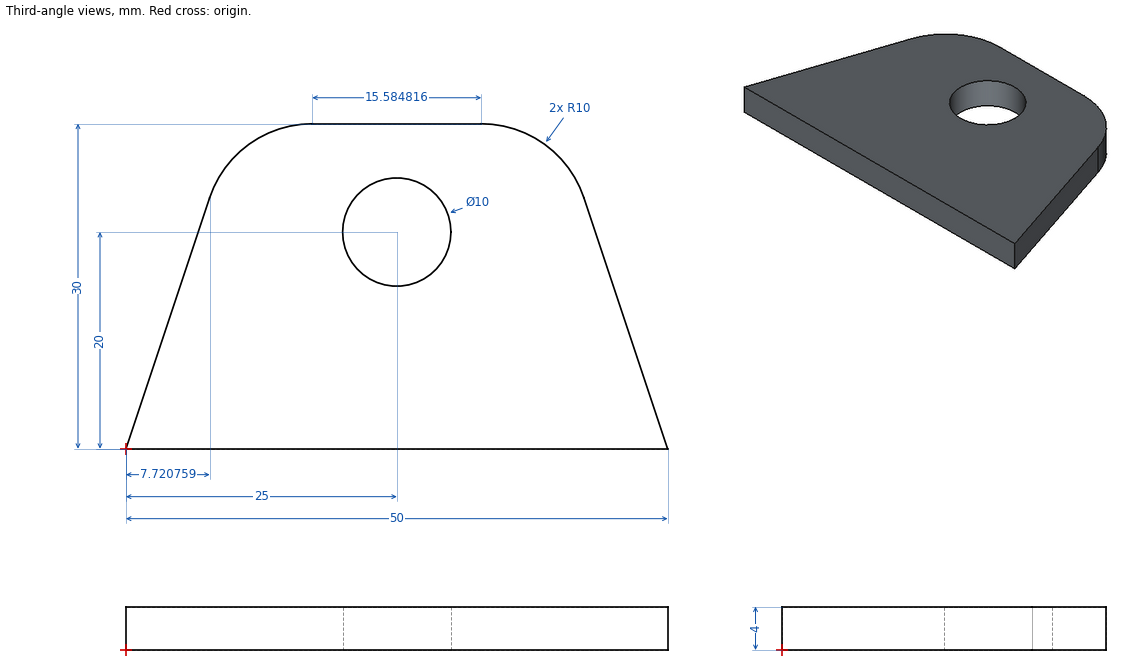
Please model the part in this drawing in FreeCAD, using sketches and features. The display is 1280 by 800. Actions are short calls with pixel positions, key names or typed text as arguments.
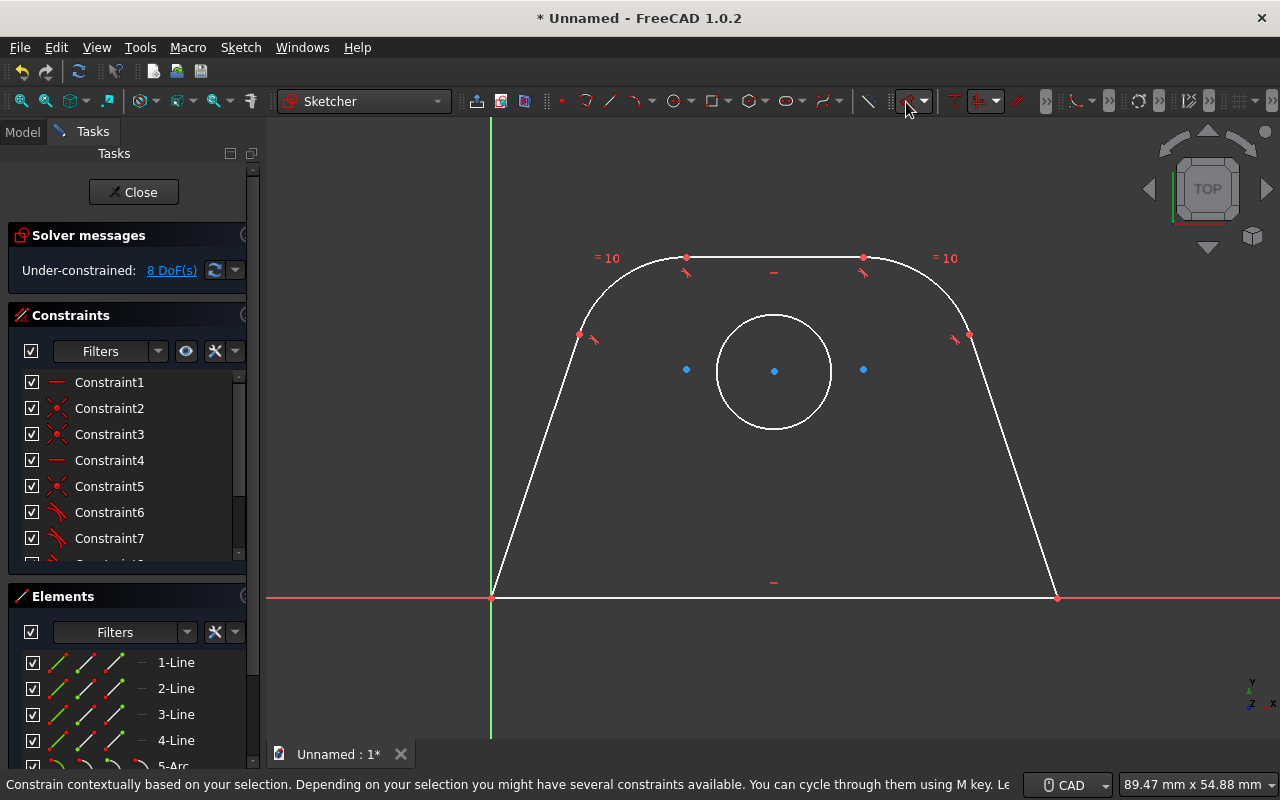
click(645, 265)
click(633, 235)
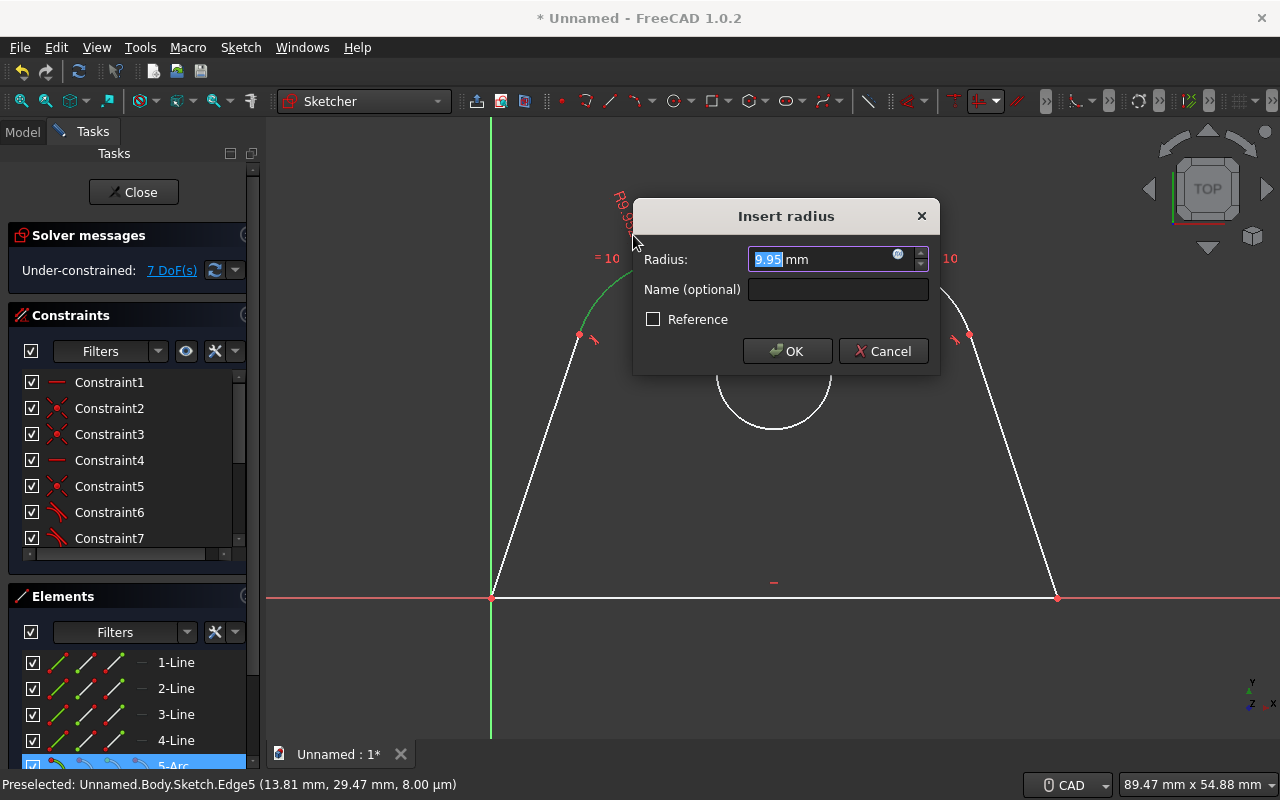
text(10)
key(Return)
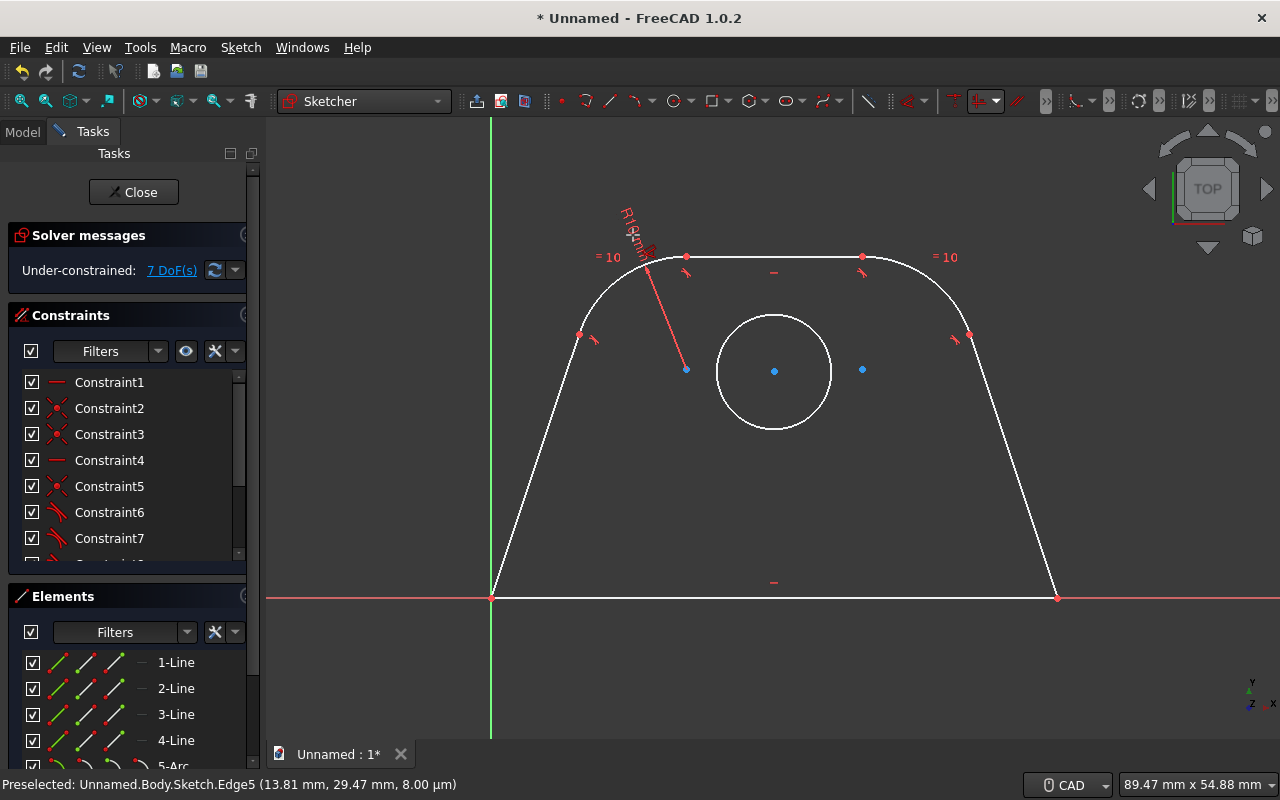
click(814, 331)
click(836, 308)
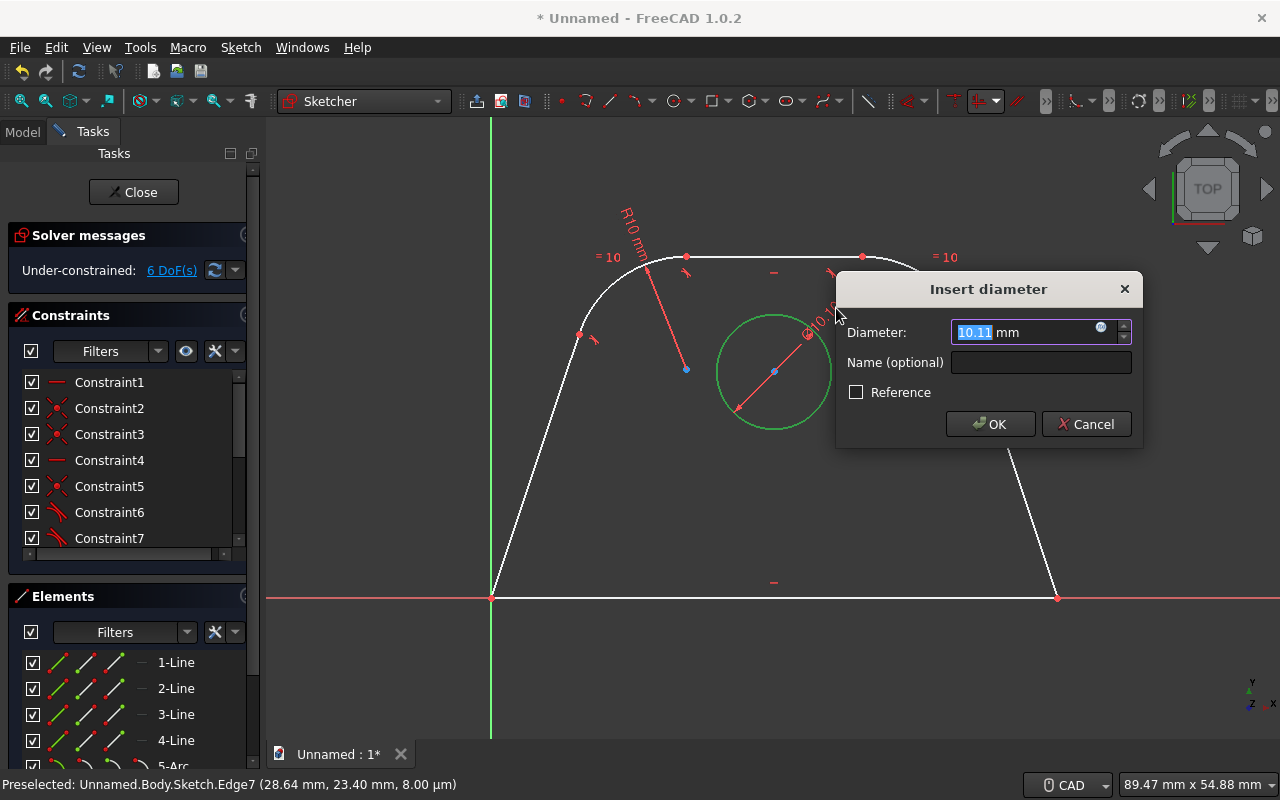
text(10)
key(Return)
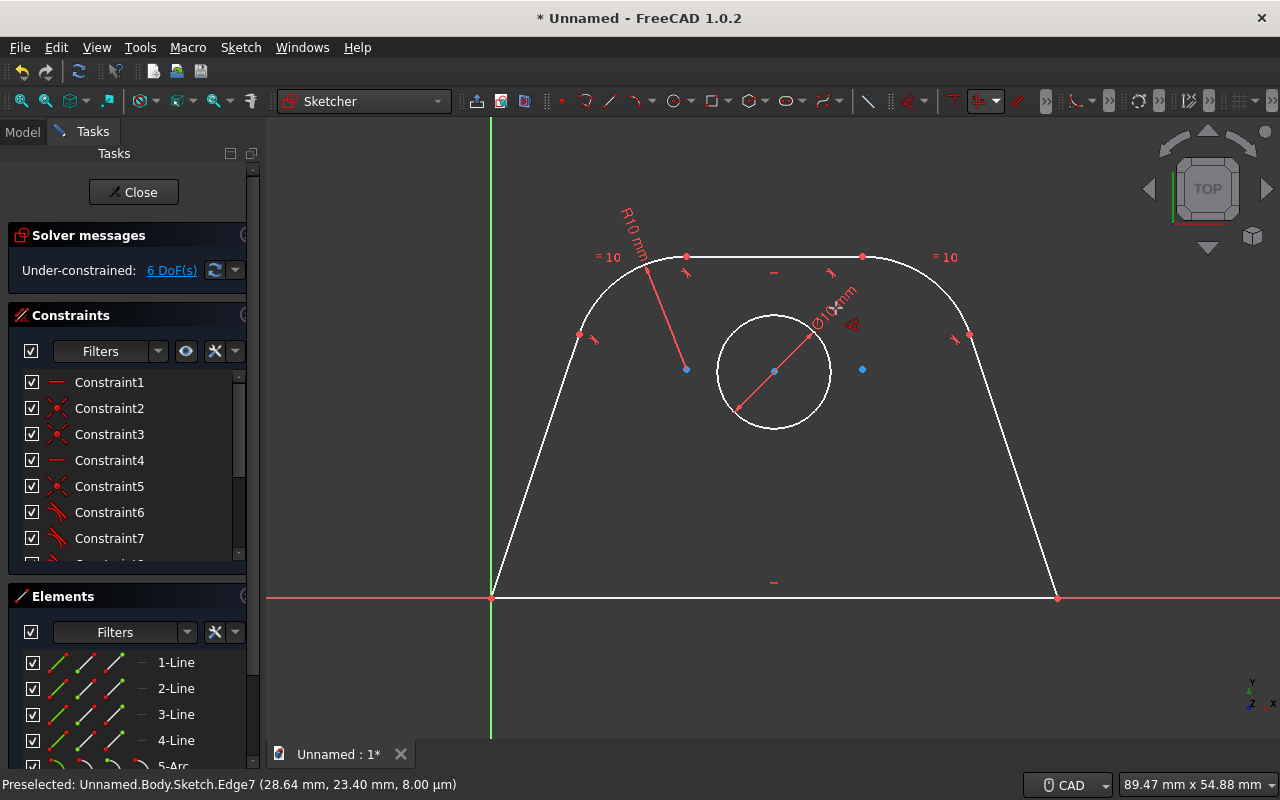
click(661, 598)
click(775, 632)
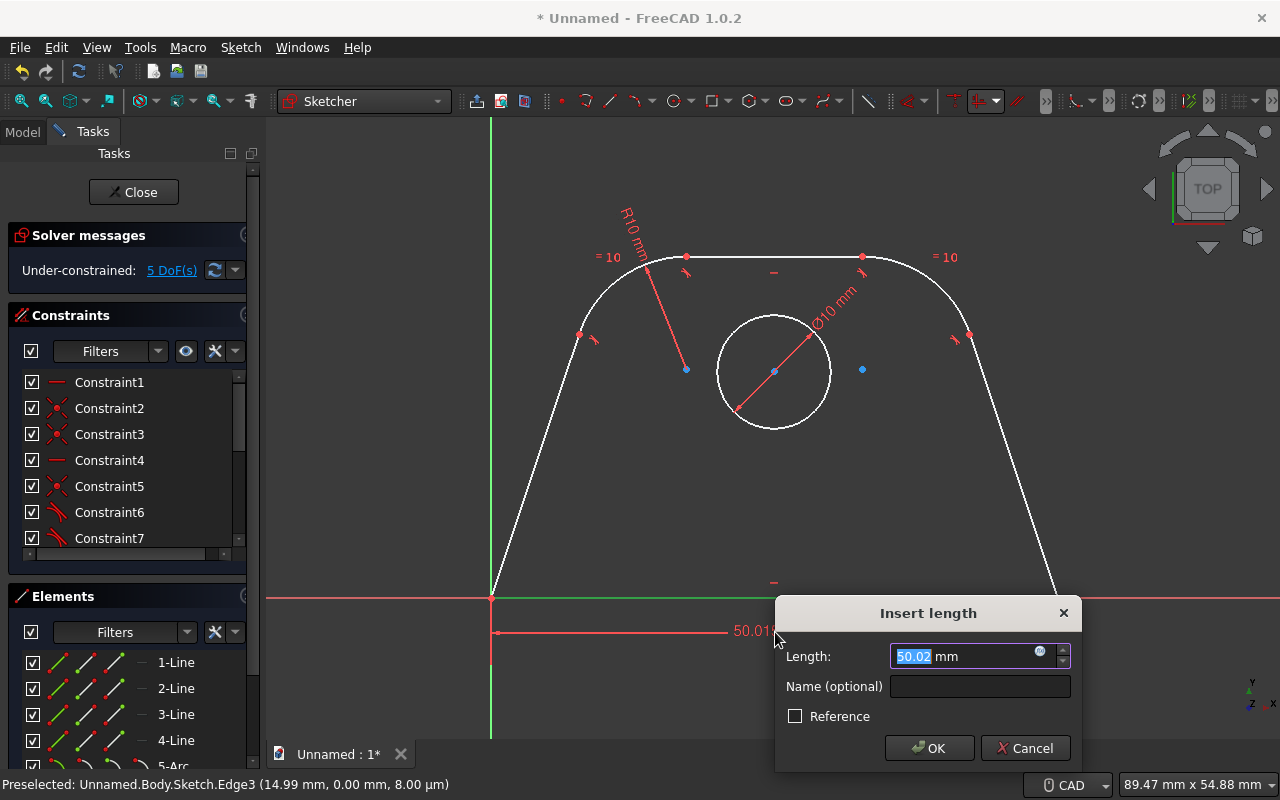
text(50)
key(Return)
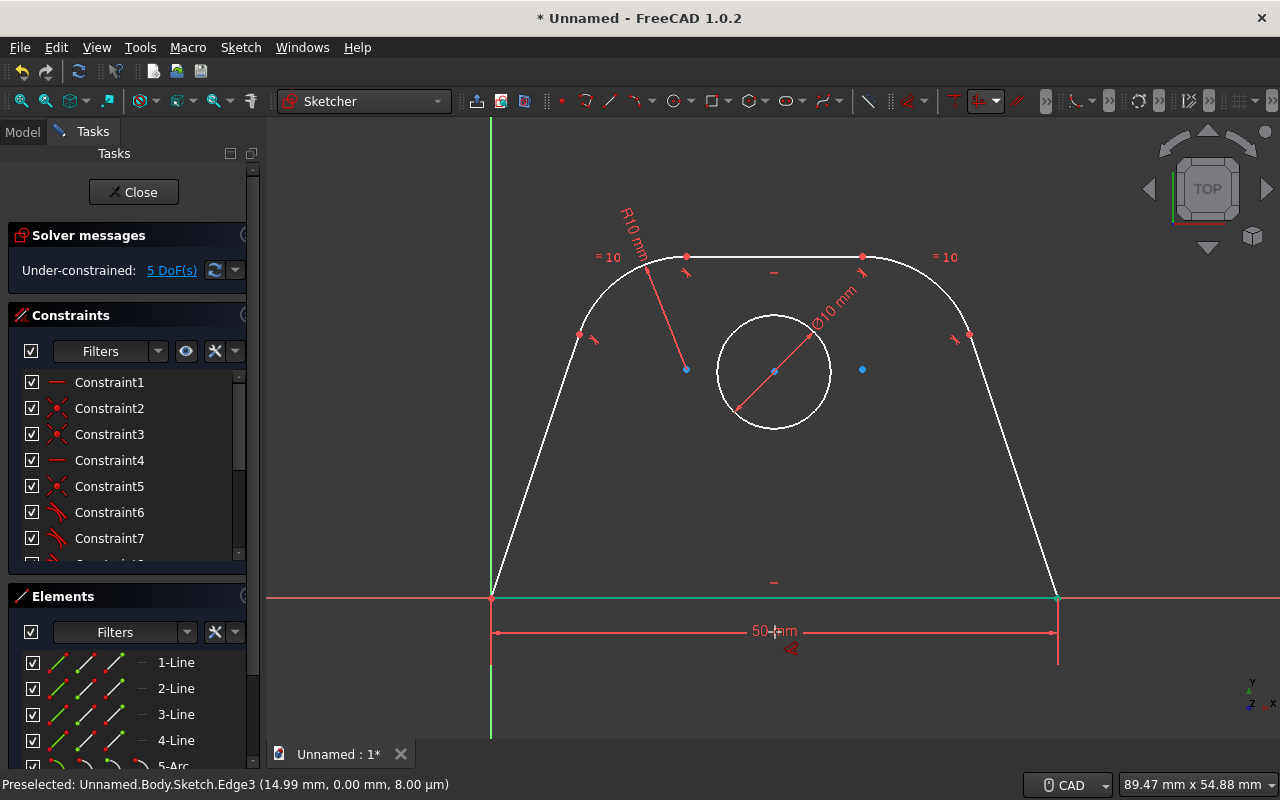
click(774, 372)
click(633, 632)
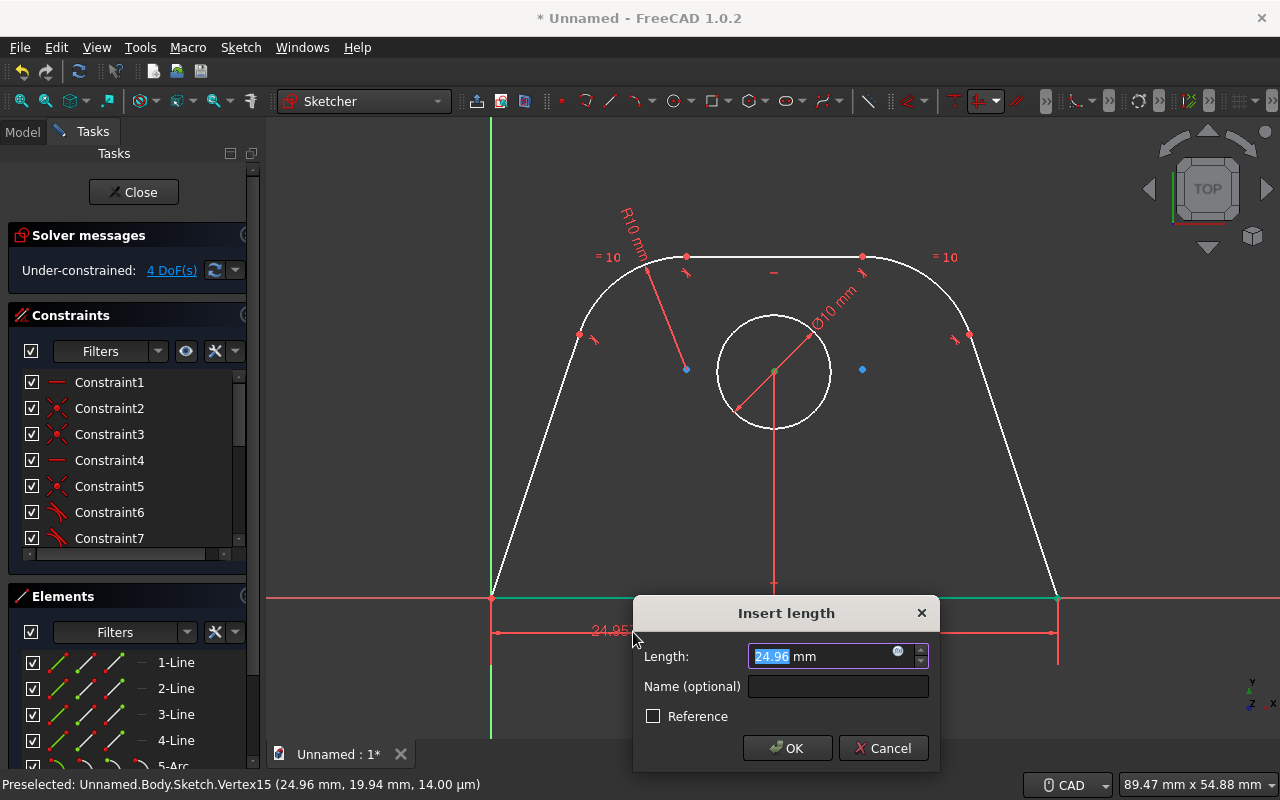
text(25)
key(Return)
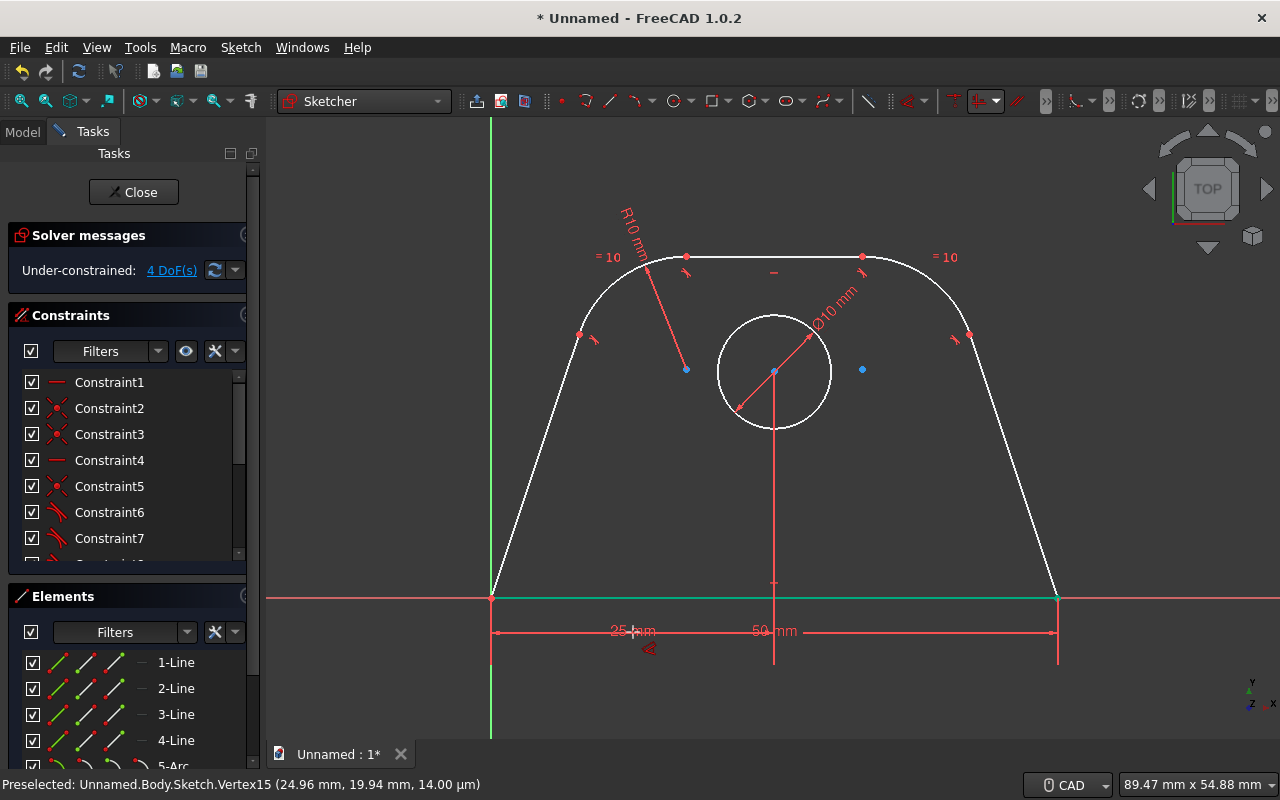
click(774, 372)
click(457, 485)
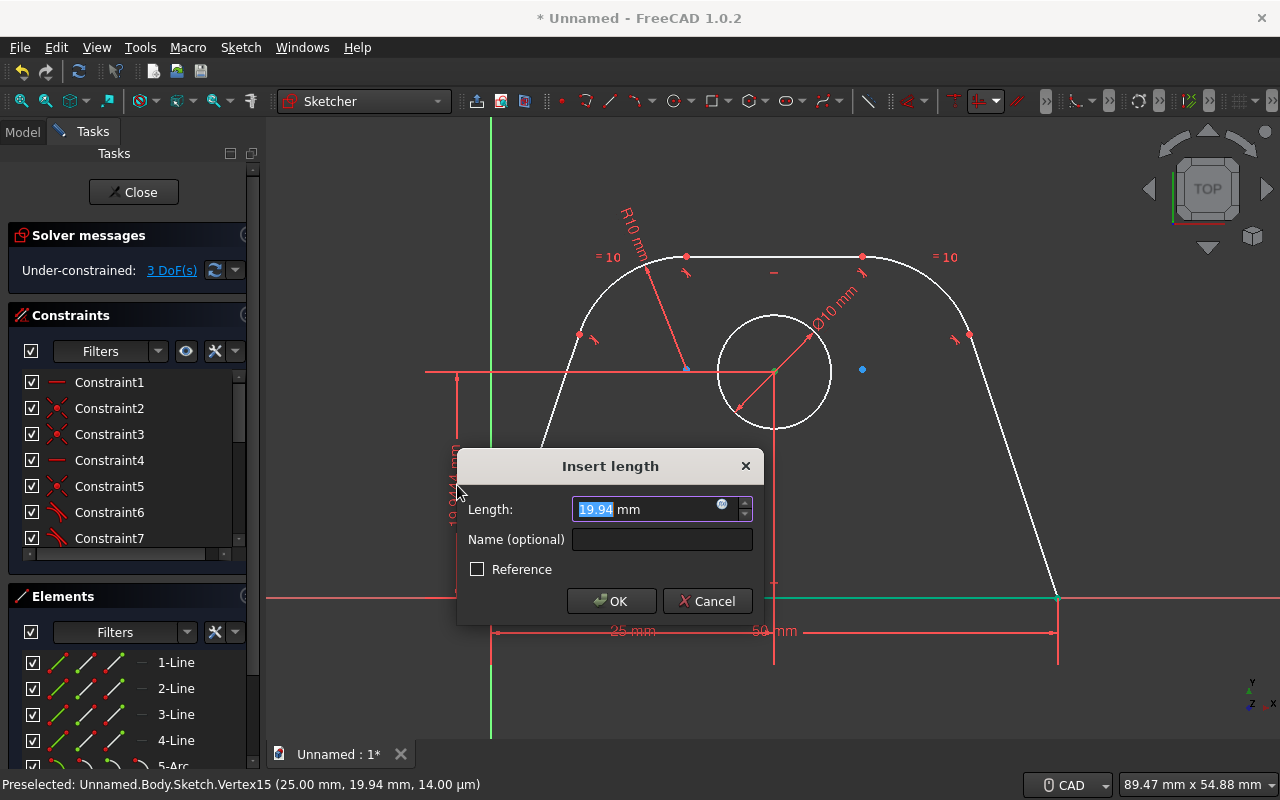
text(20)
key(Return)